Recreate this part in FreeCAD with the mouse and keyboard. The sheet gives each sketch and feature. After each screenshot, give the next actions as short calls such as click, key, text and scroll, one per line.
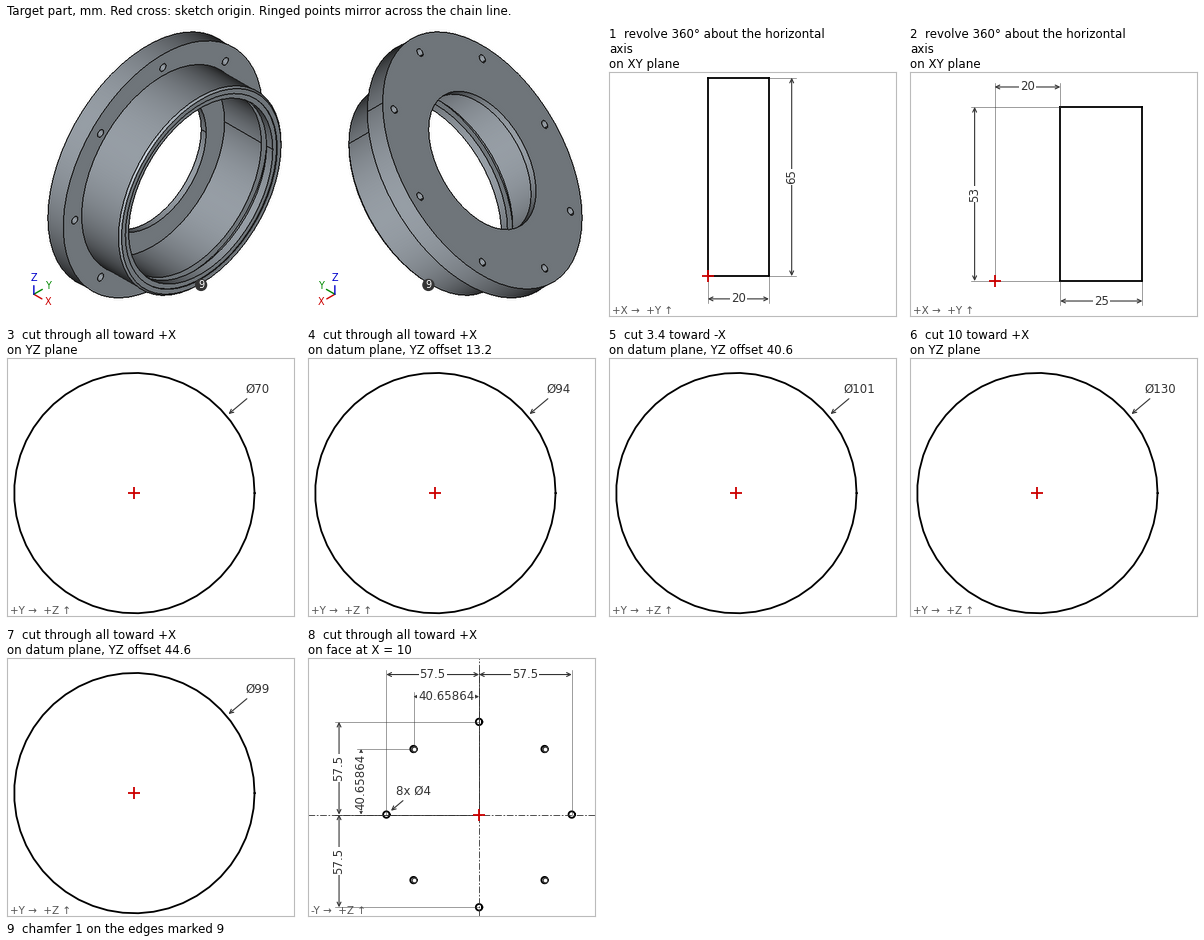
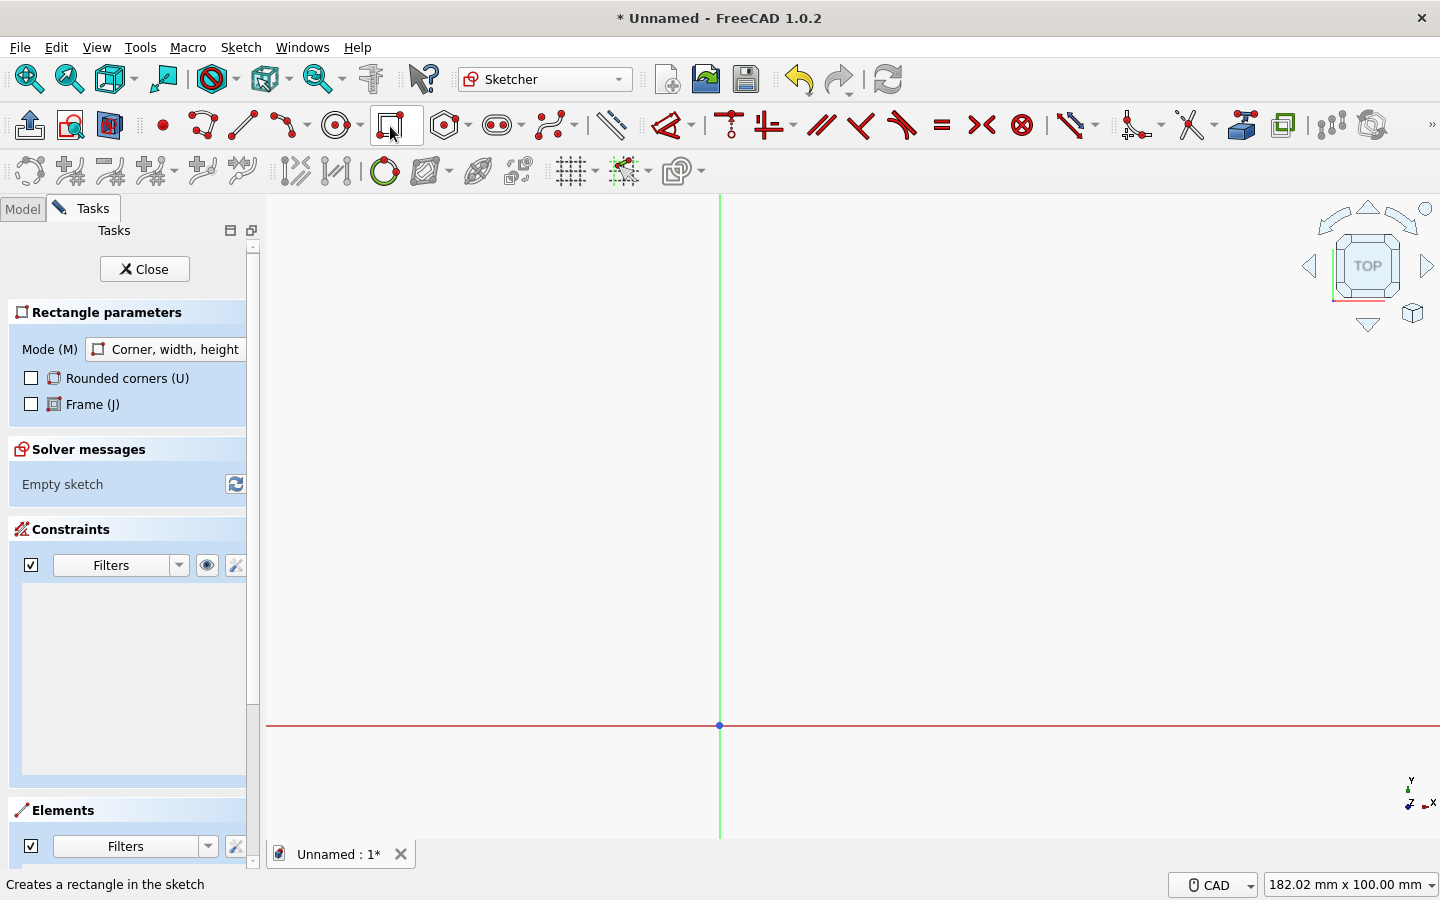
click(720, 726)
click(849, 307)
key(Escape)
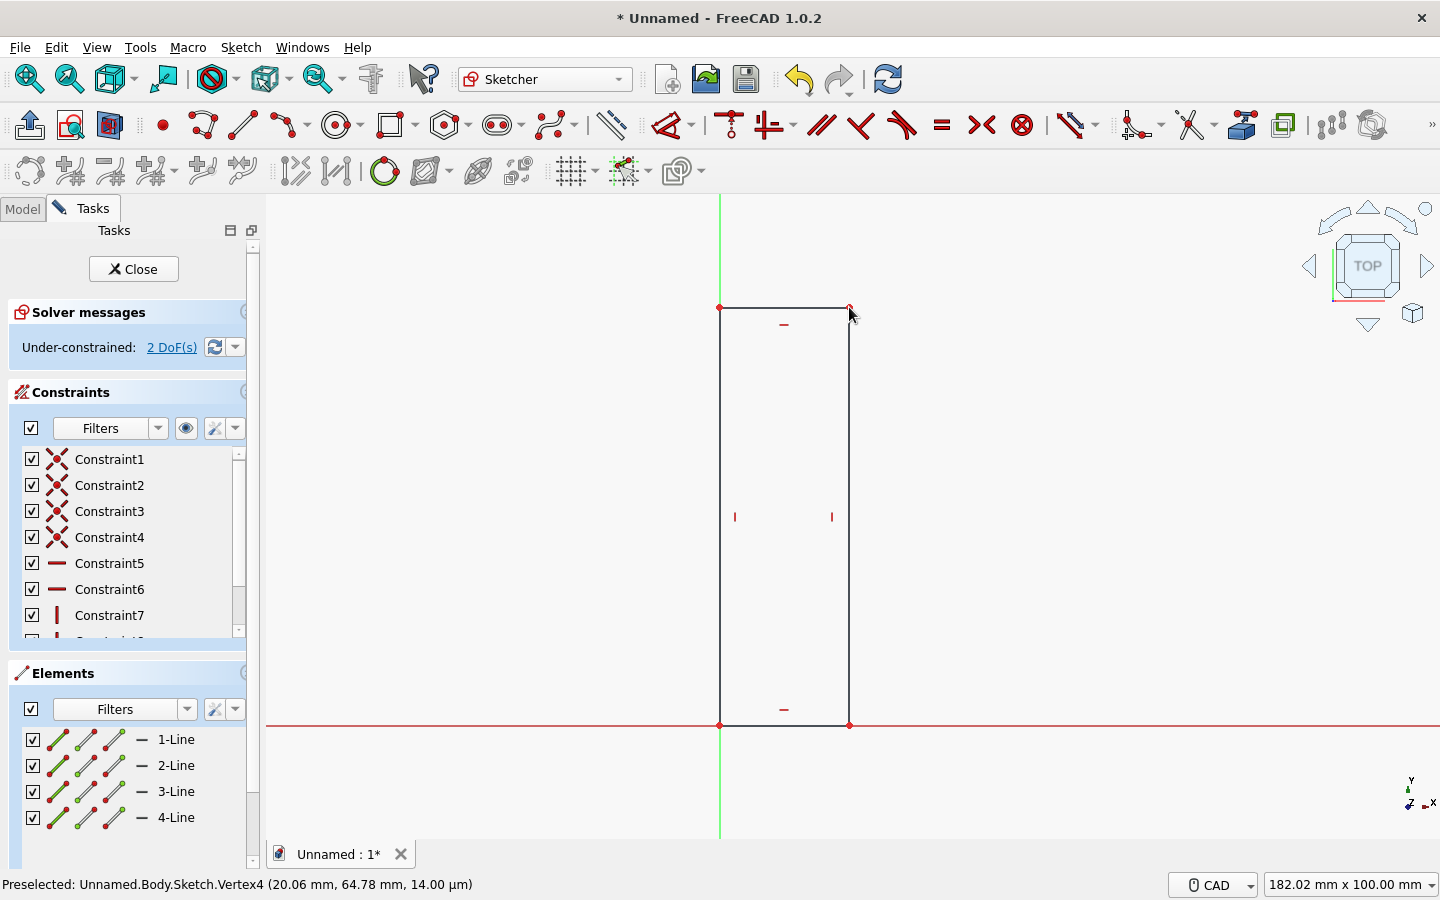
click(666, 126)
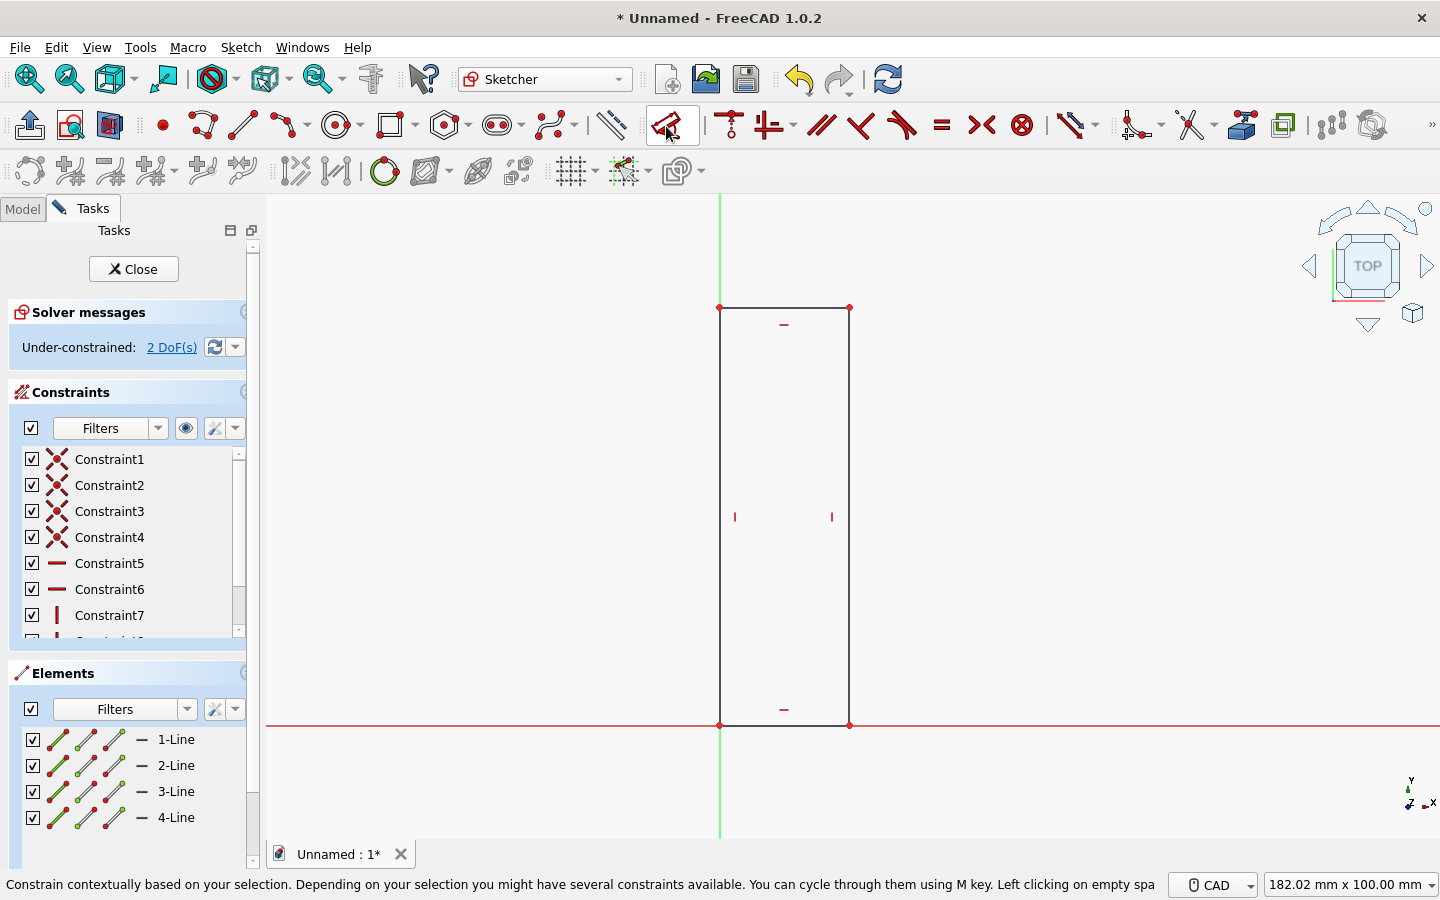
click(758, 726)
click(784, 760)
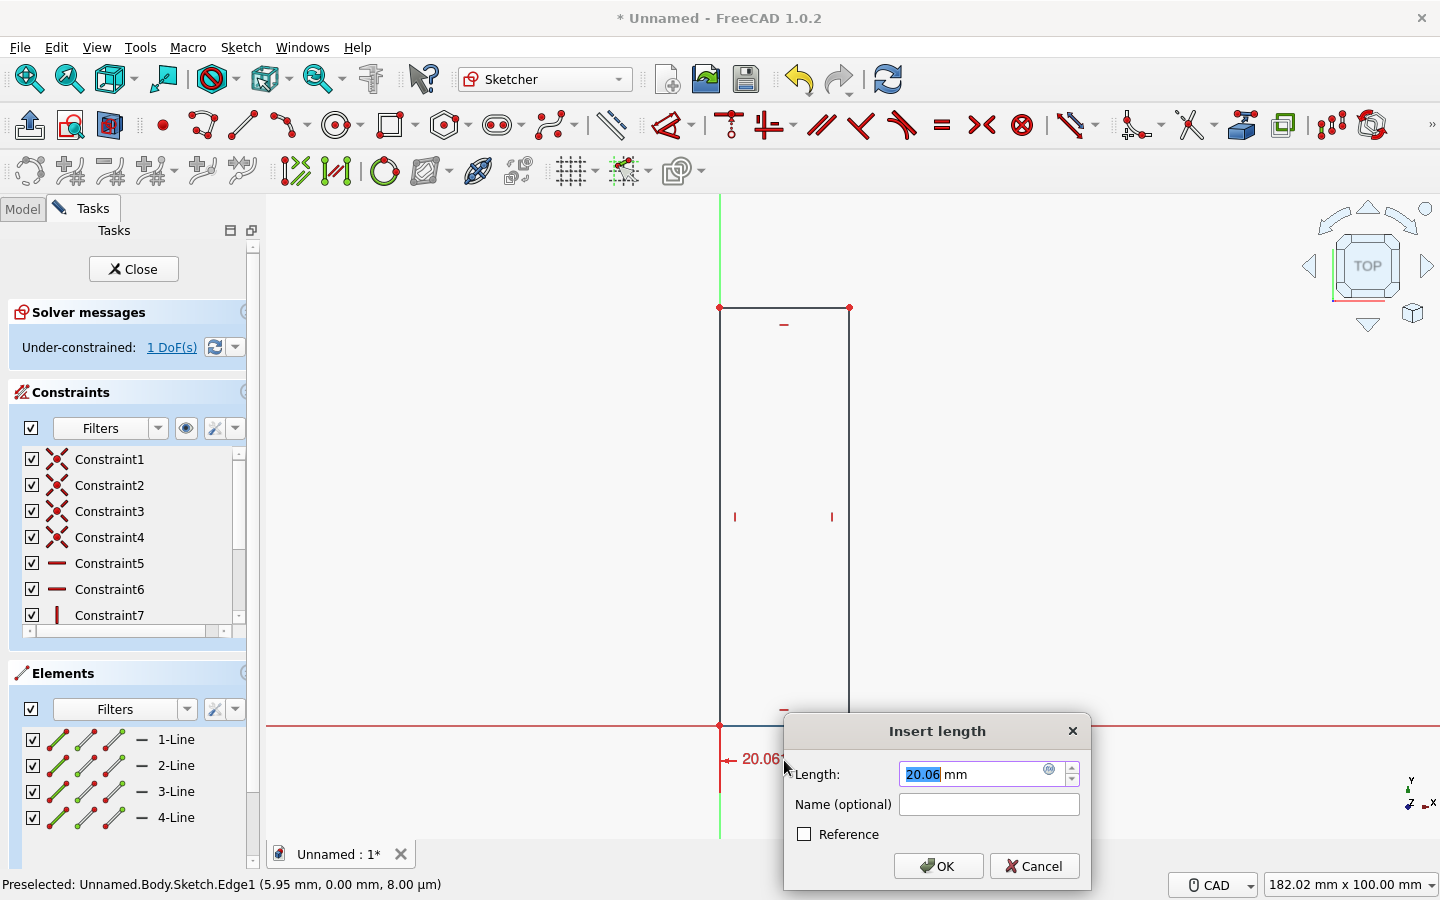
text(20)
key(Return)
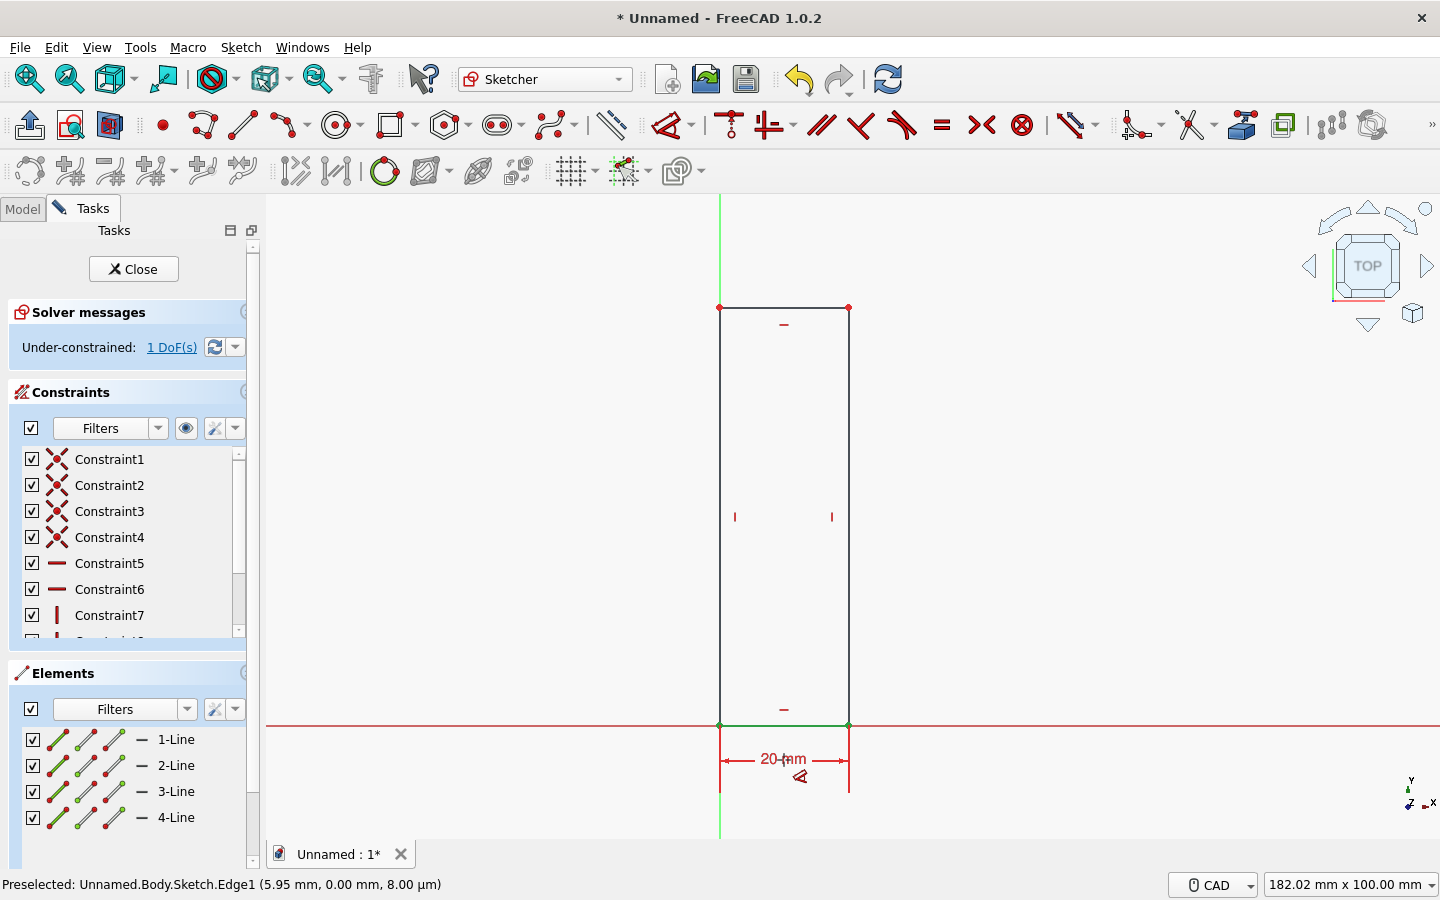
click(849, 600)
click(883, 517)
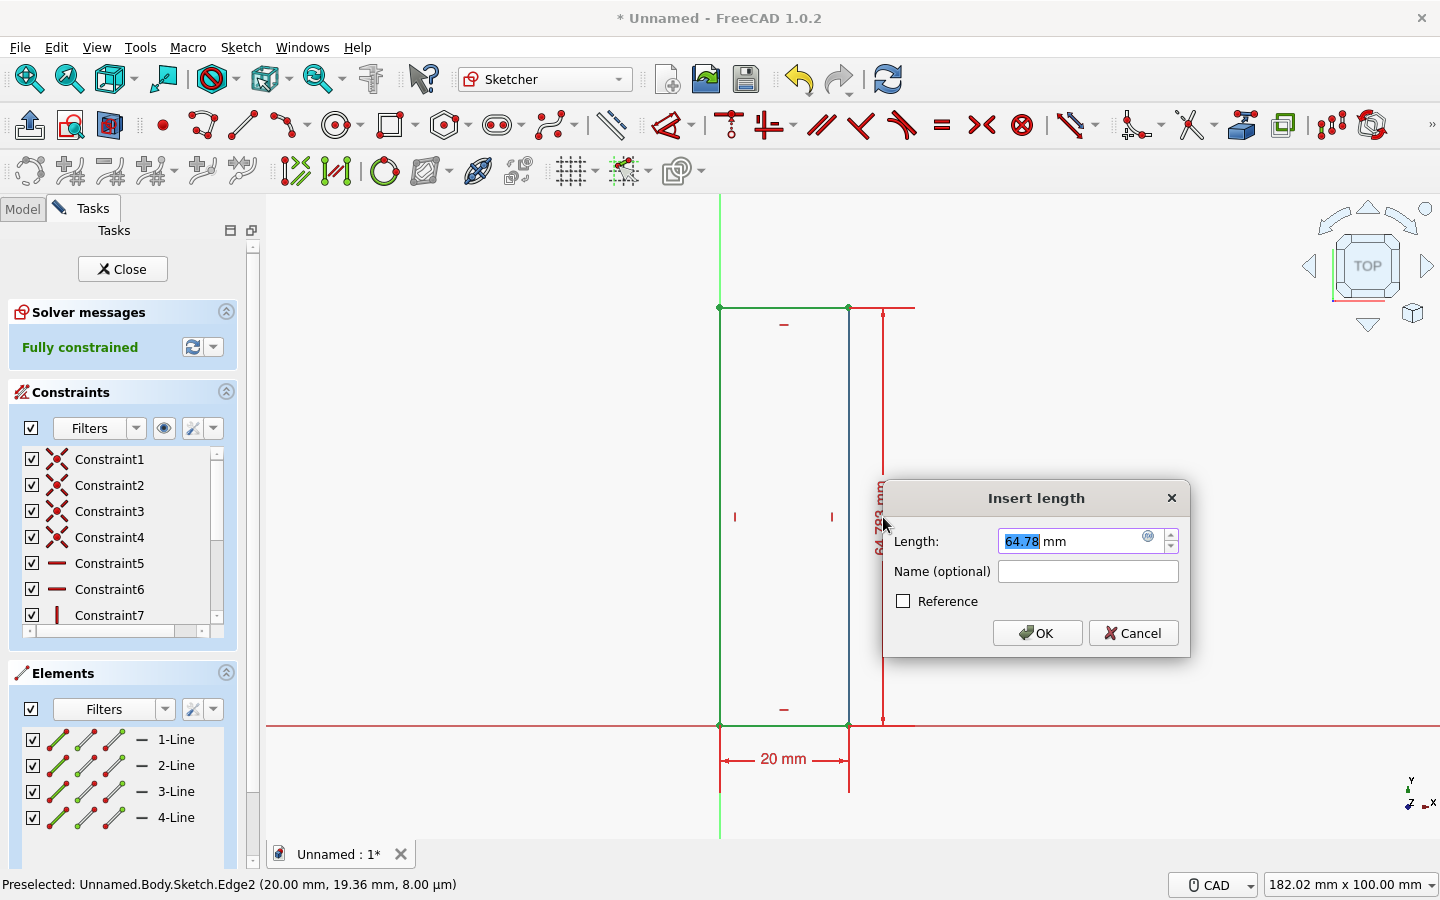
text(65)
key(Return)
key(Escape)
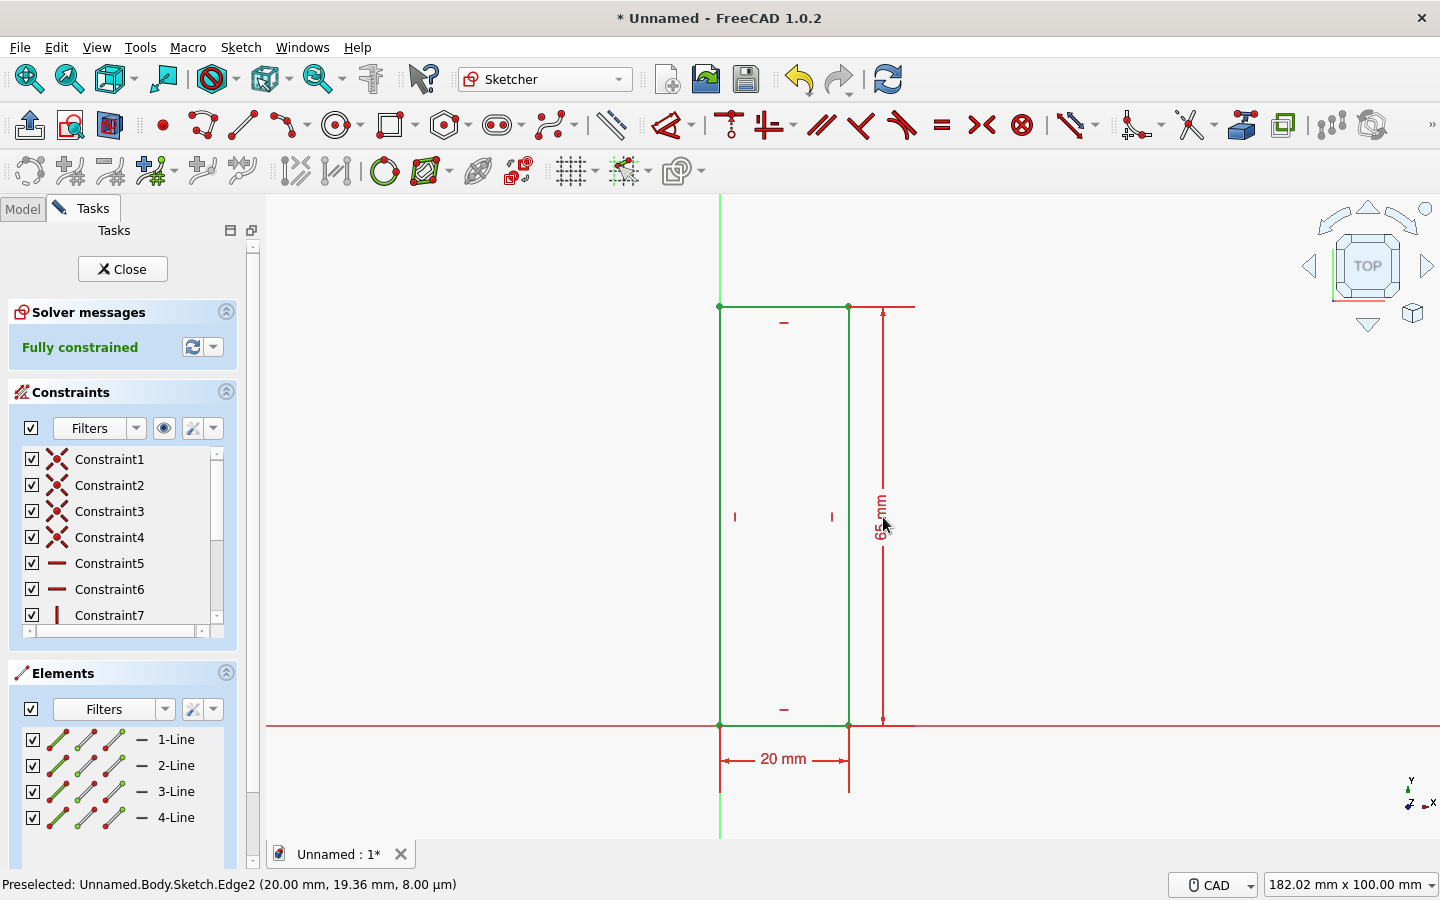
click(123, 269)